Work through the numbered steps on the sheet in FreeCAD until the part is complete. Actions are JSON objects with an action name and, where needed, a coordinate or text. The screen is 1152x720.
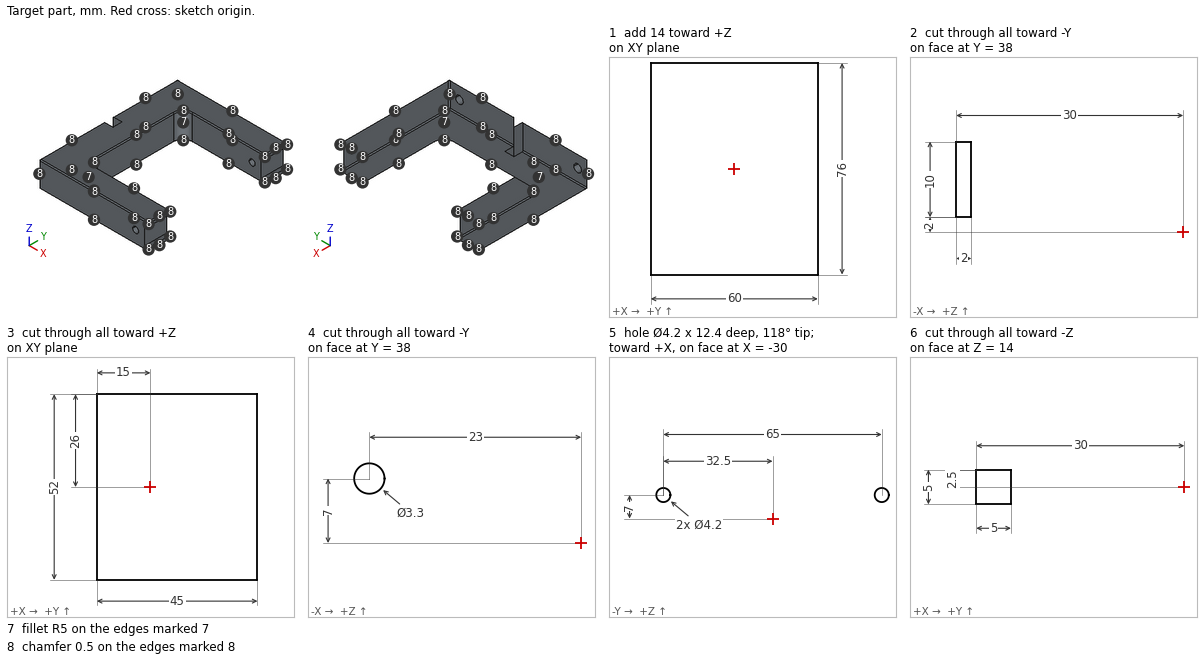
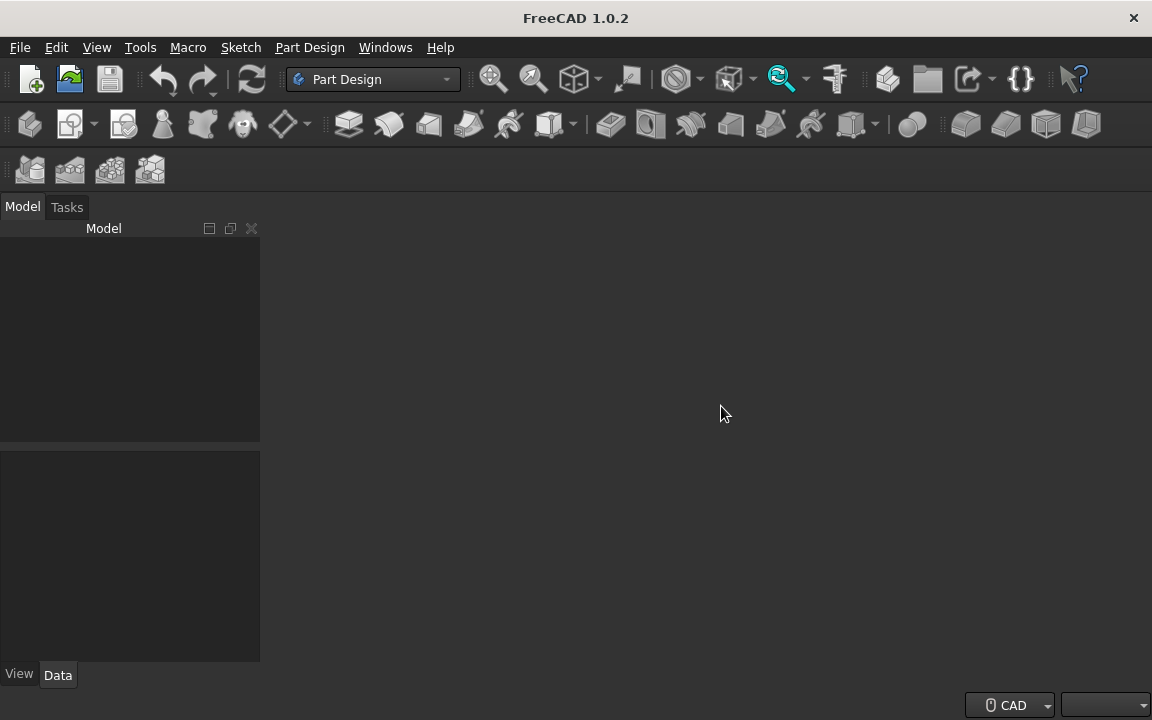
{"action": "key", "text": "ctrl+n"}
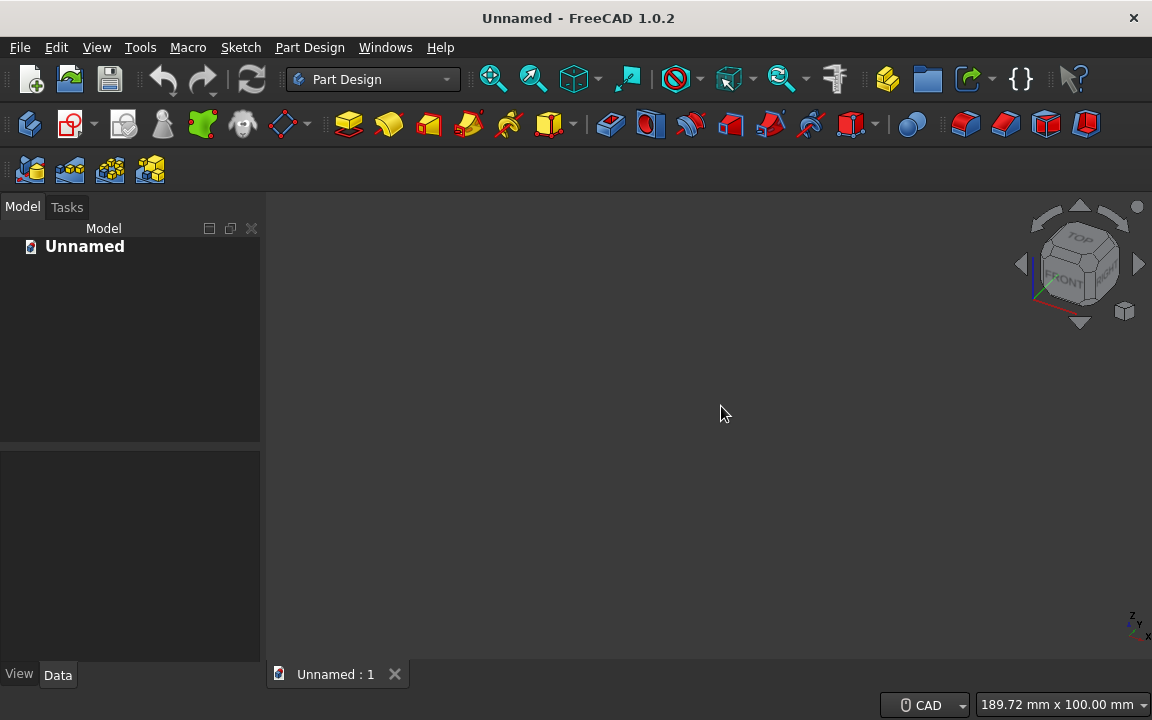
{"action": "left_click", "coordinate": [70, 124]}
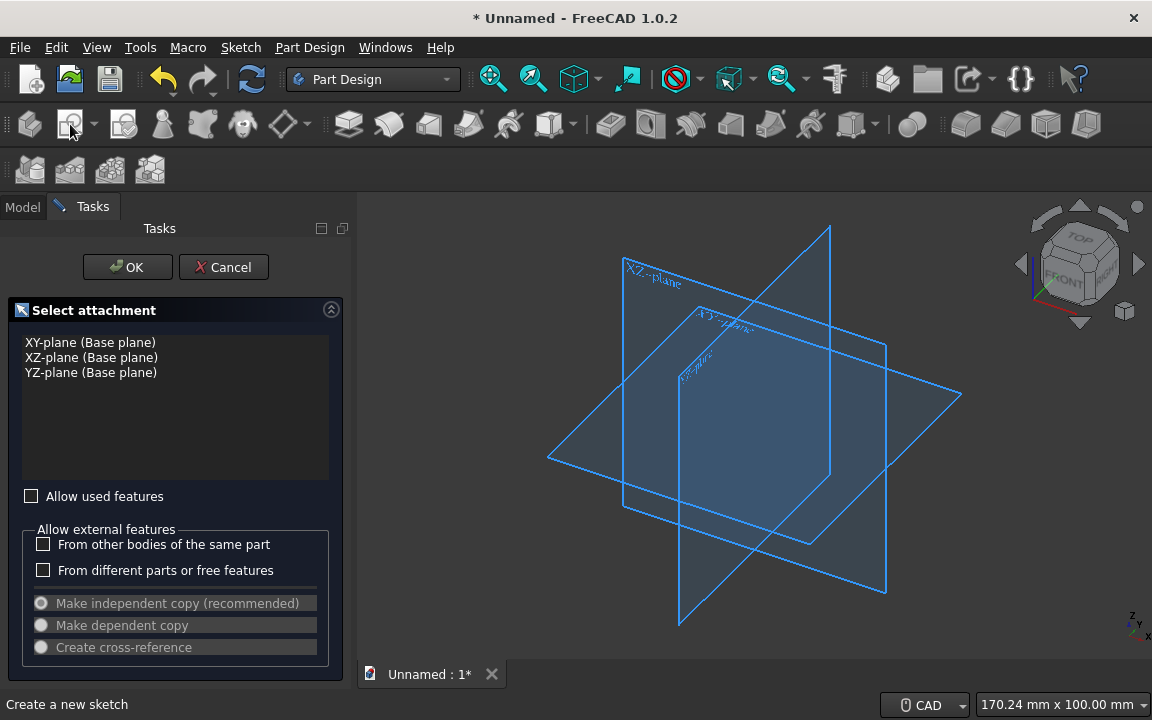
{"action": "left_click", "coordinate": [82, 342]}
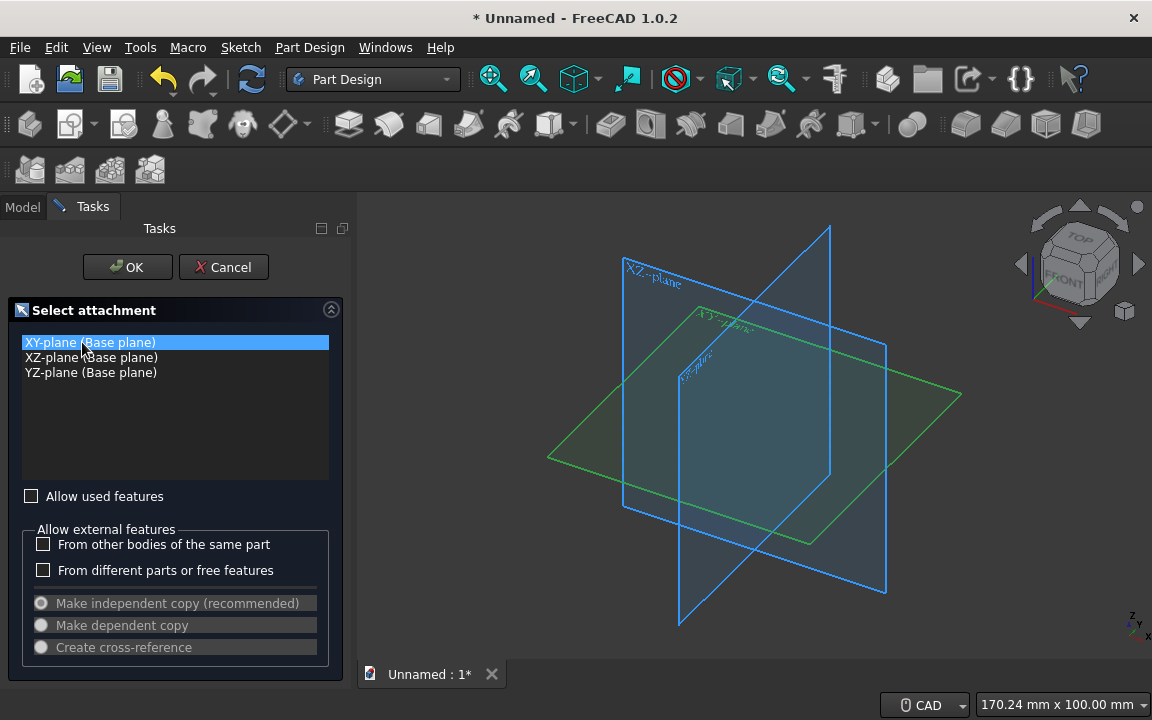
{"action": "left_click", "coordinate": [128, 267]}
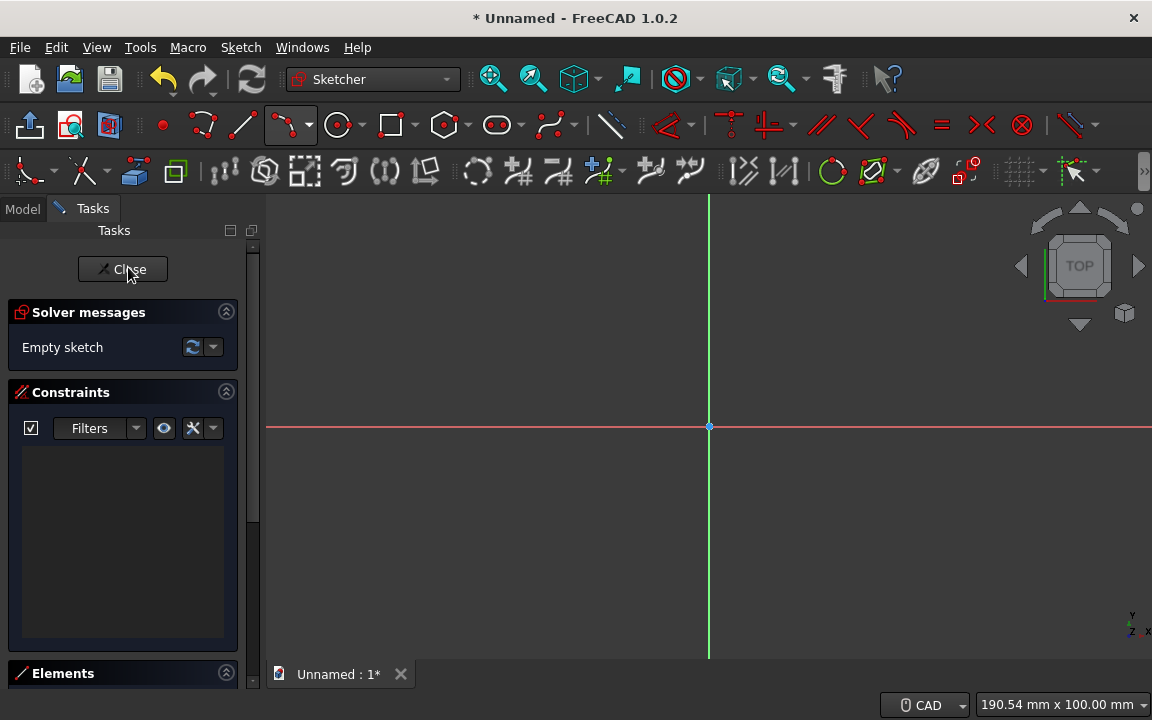
{"action": "key", "text": "g v"}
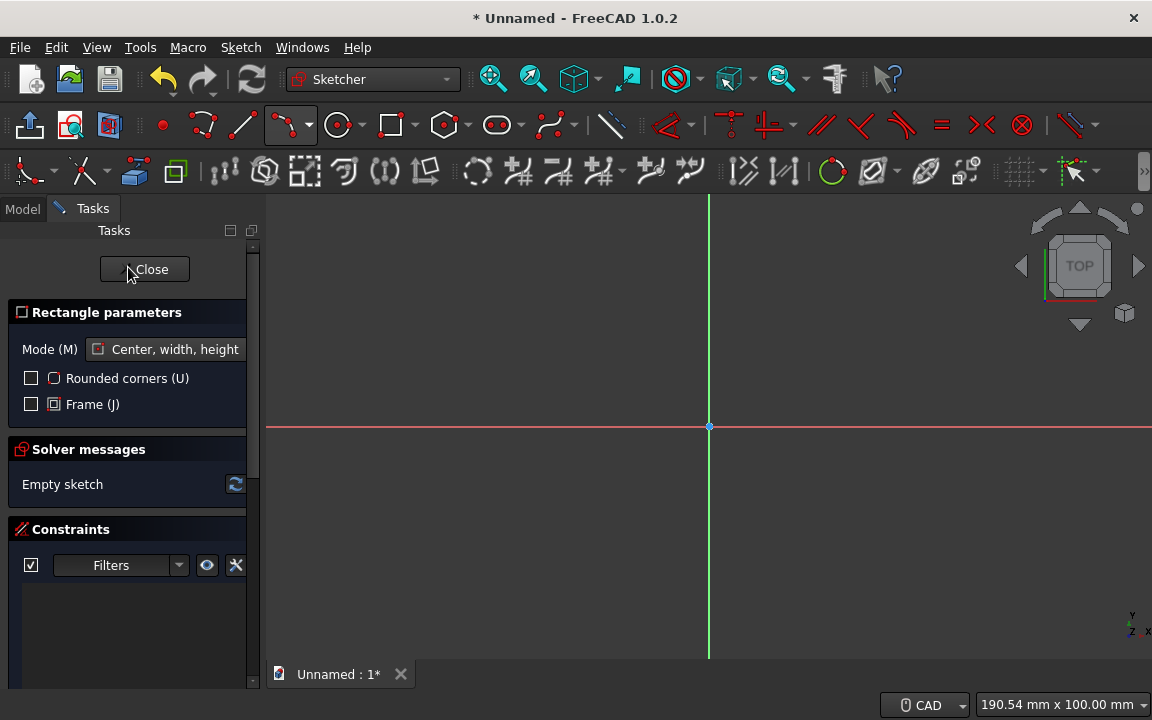
{"action": "left_click", "coordinate": [709, 426]}
{"action": "left_click", "coordinate": [848, 250]}
{"action": "key", "text": "Escape"}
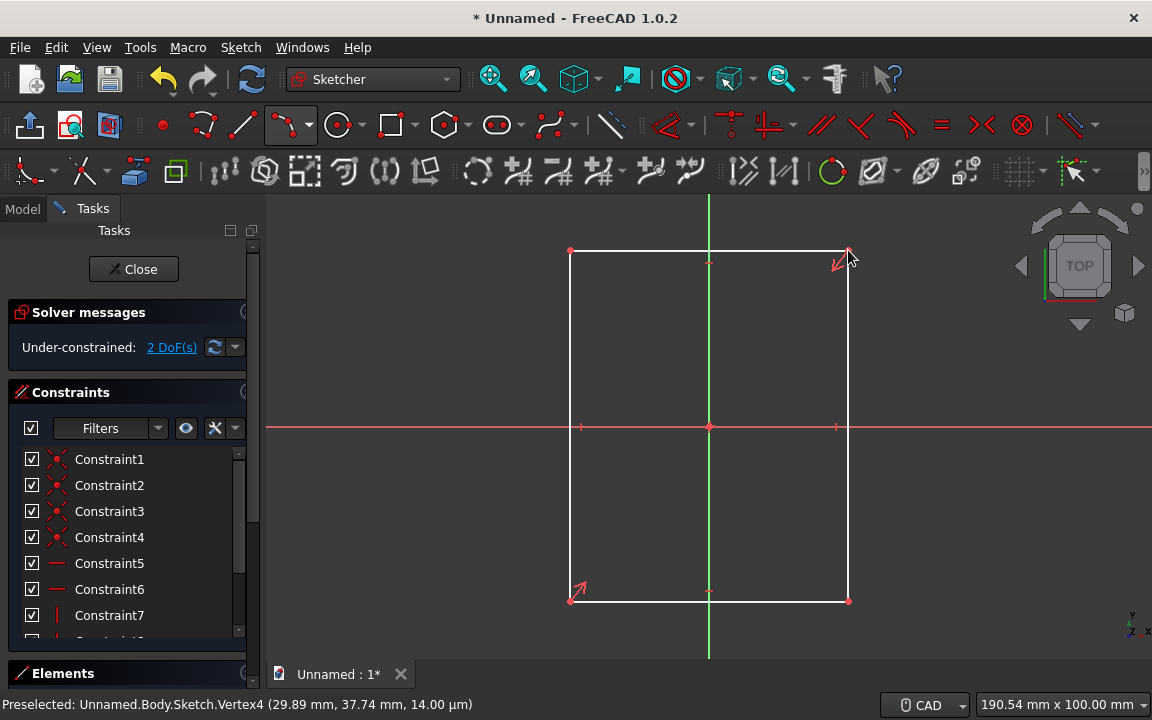
{"action": "left_click", "coordinate": [653, 602]}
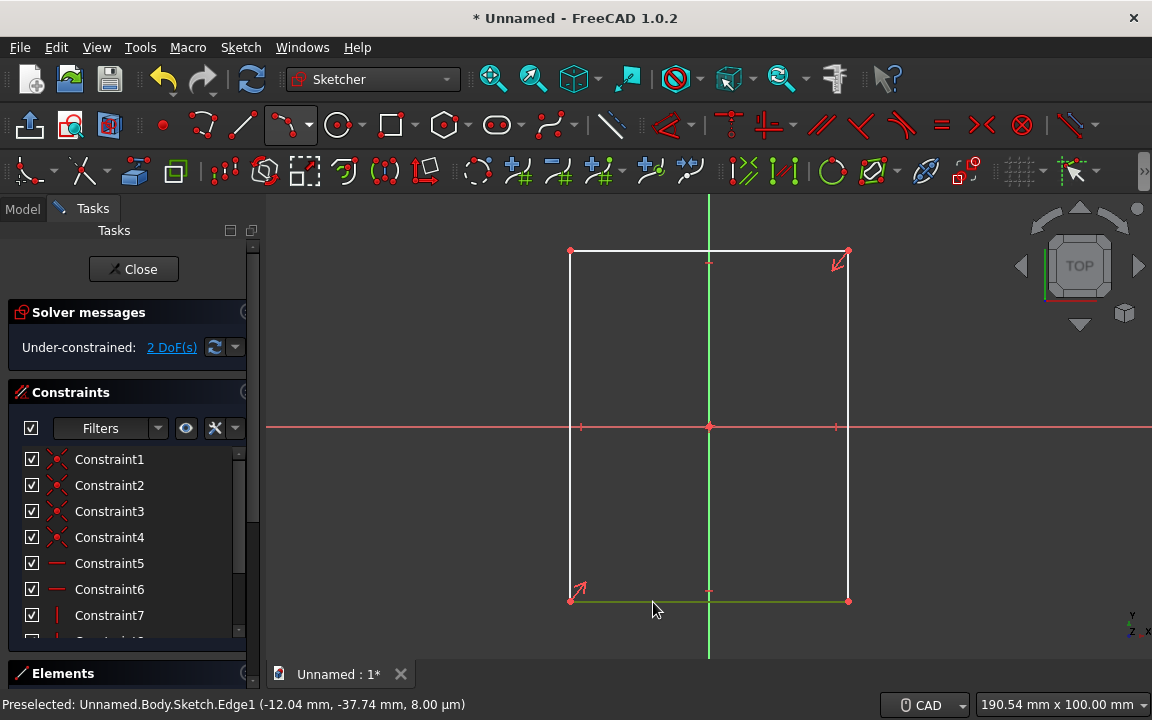
{"action": "key", "text": "l"}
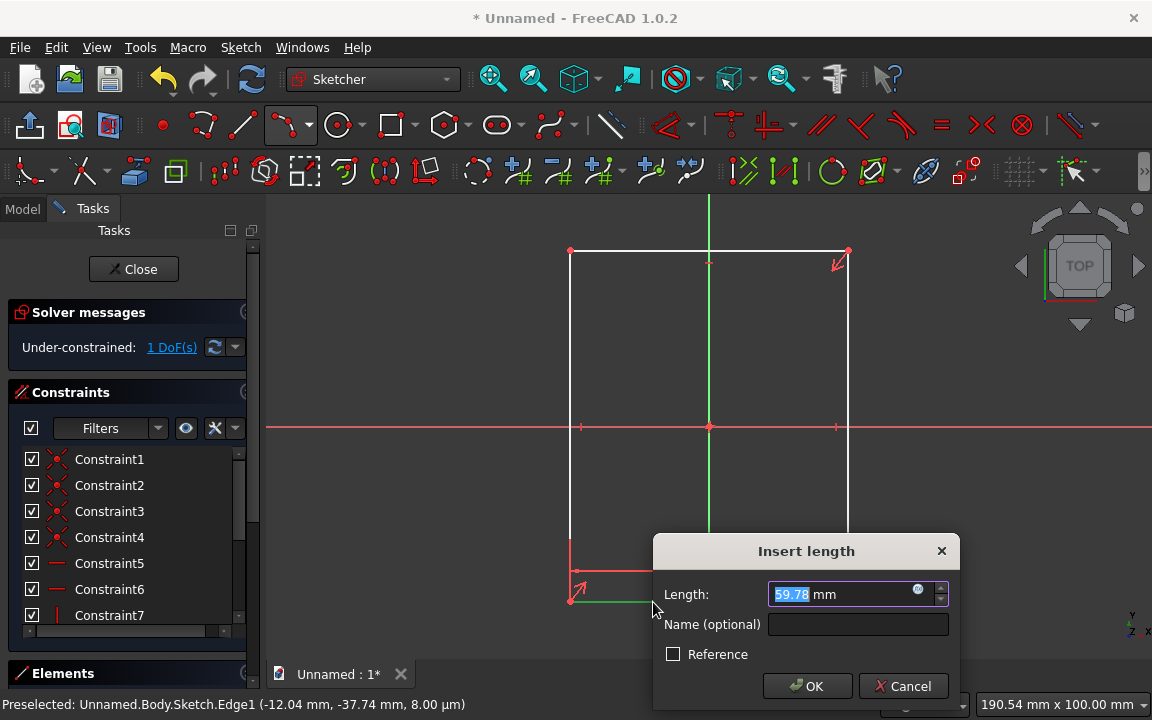
{"action": "type", "text": "60"}
{"action": "key", "text": "Return"}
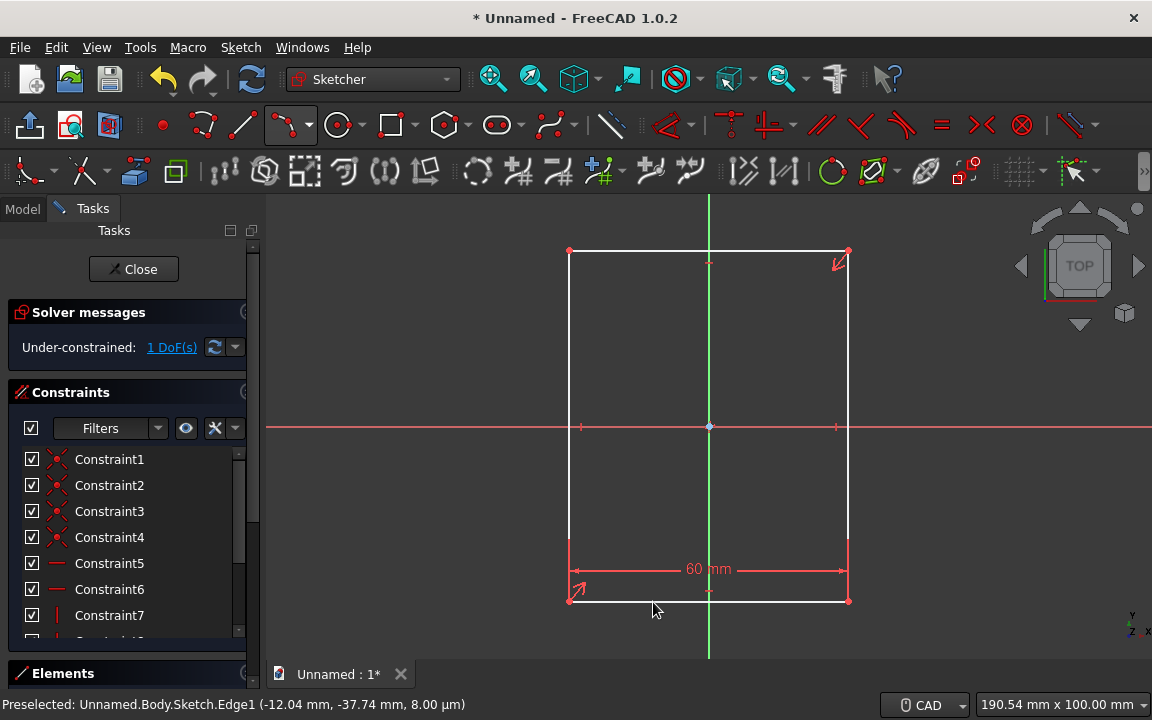
{"action": "left_click", "coordinate": [848, 497]}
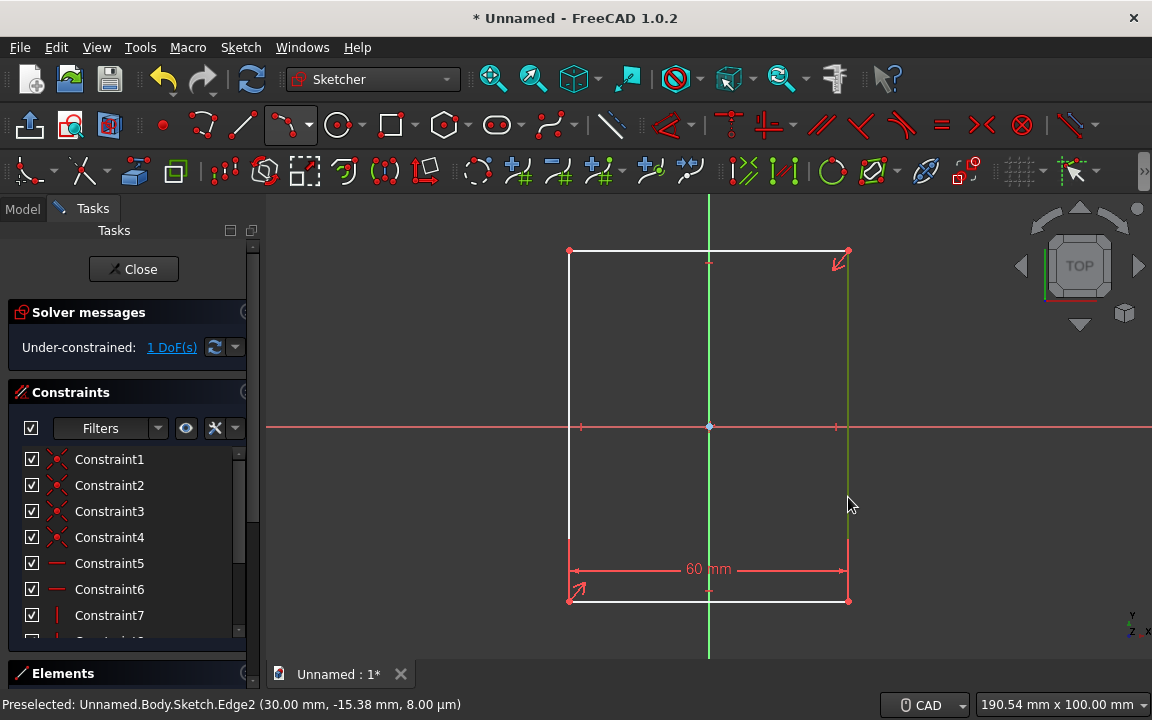
{"action": "left_click", "coordinate": [694, 126]}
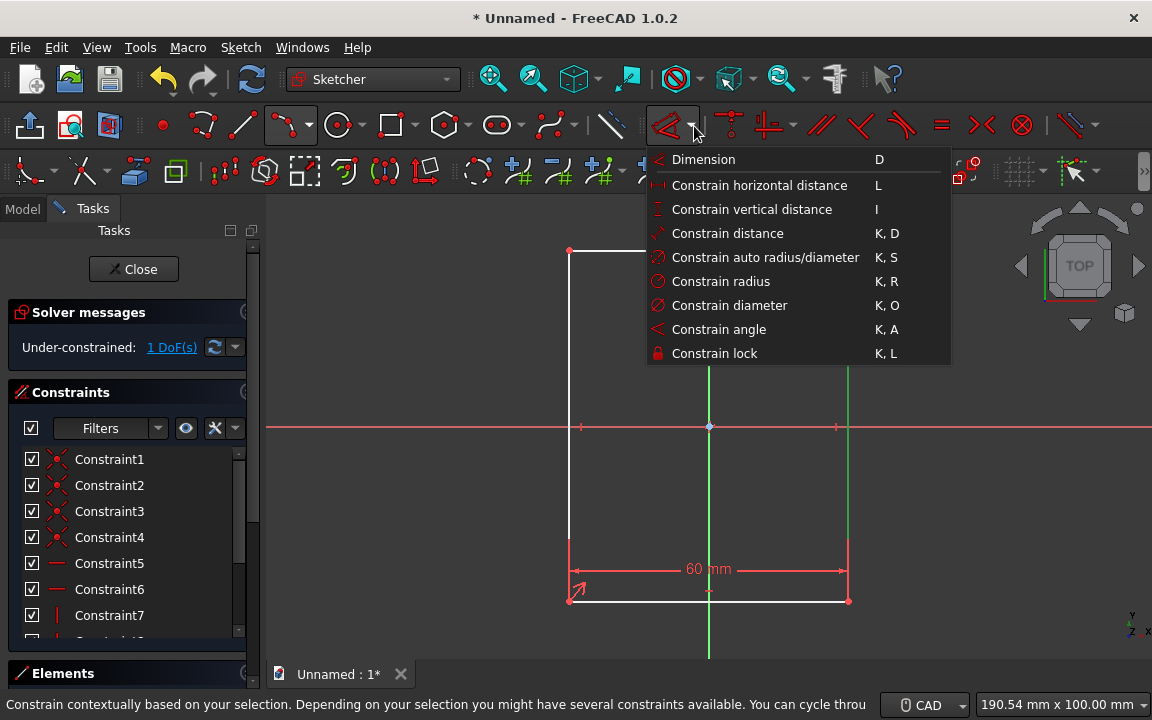
{"action": "left_click", "coordinate": [799, 209]}